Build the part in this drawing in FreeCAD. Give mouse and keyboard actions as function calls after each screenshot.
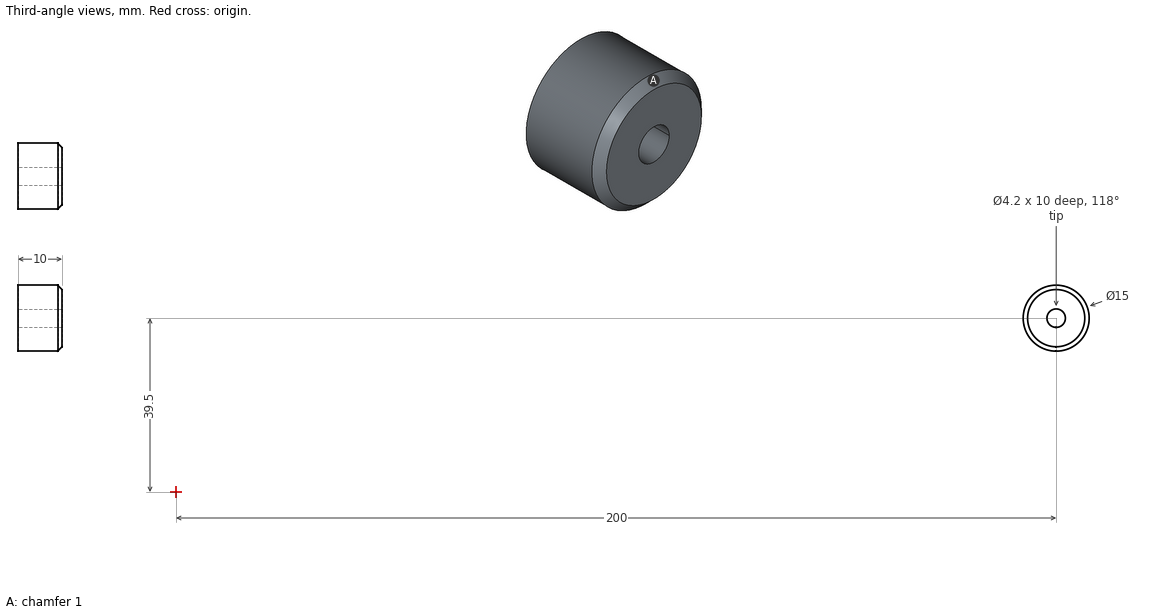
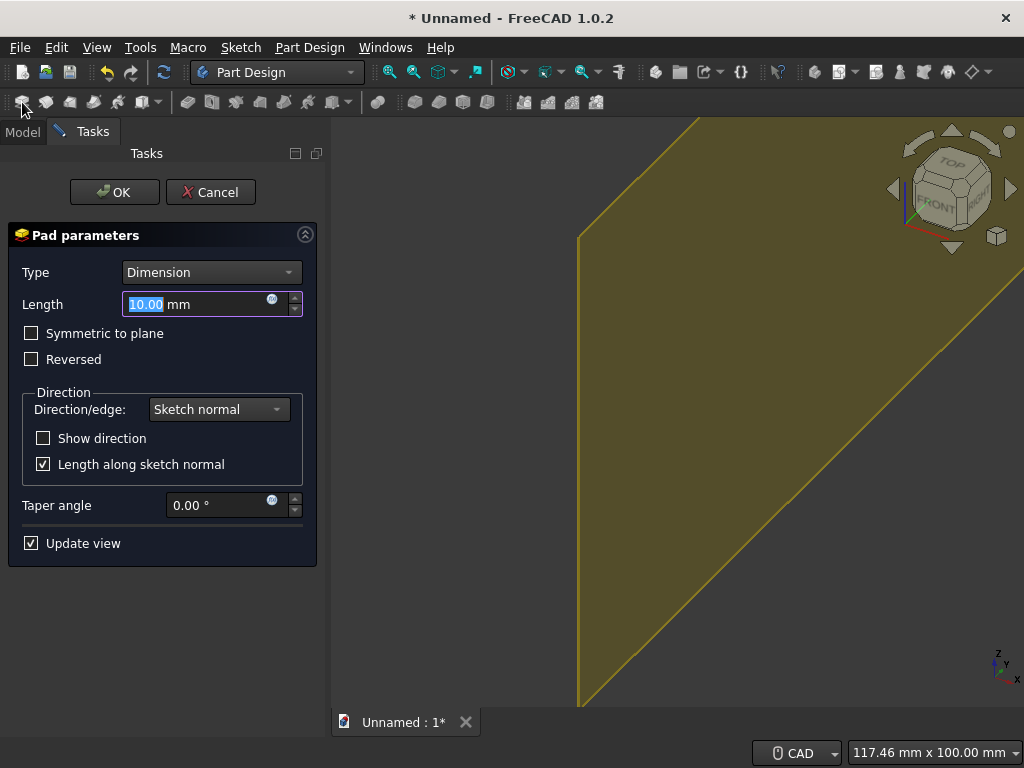
text(10)
key(Tab)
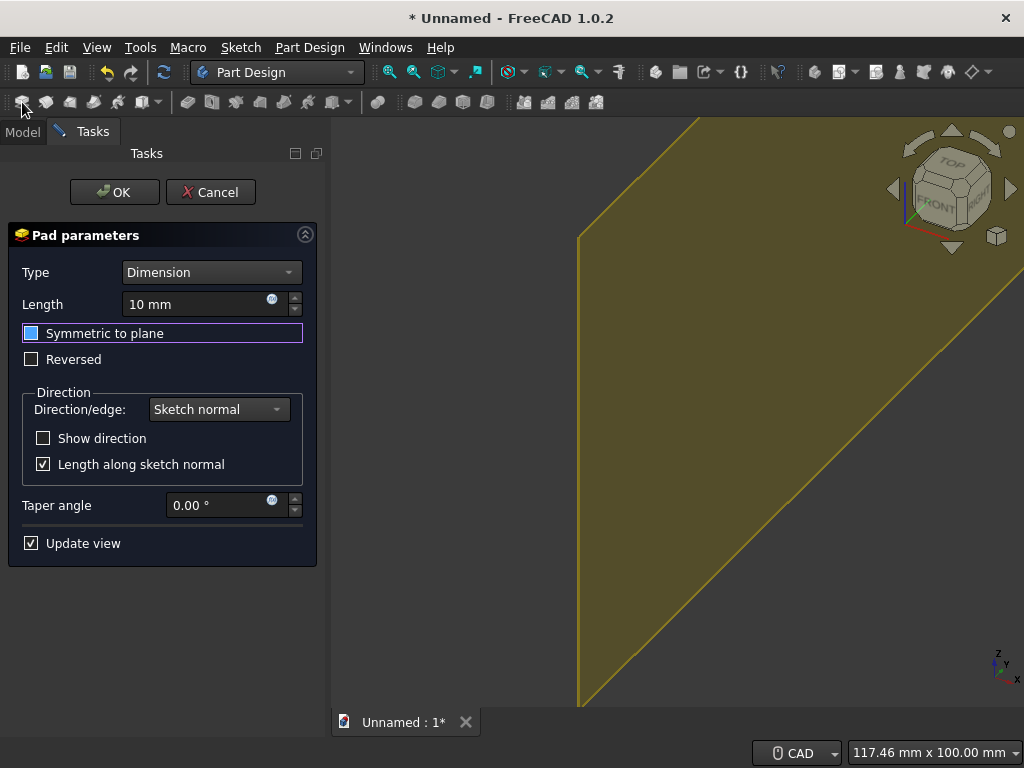
click(115, 192)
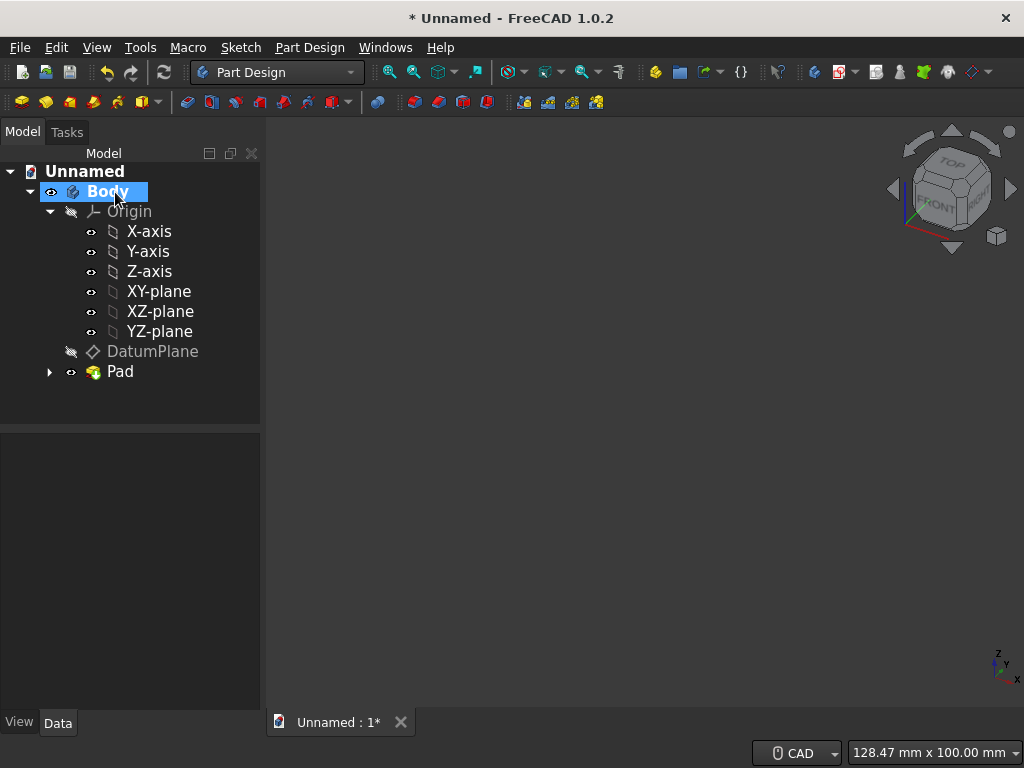
click(390, 72)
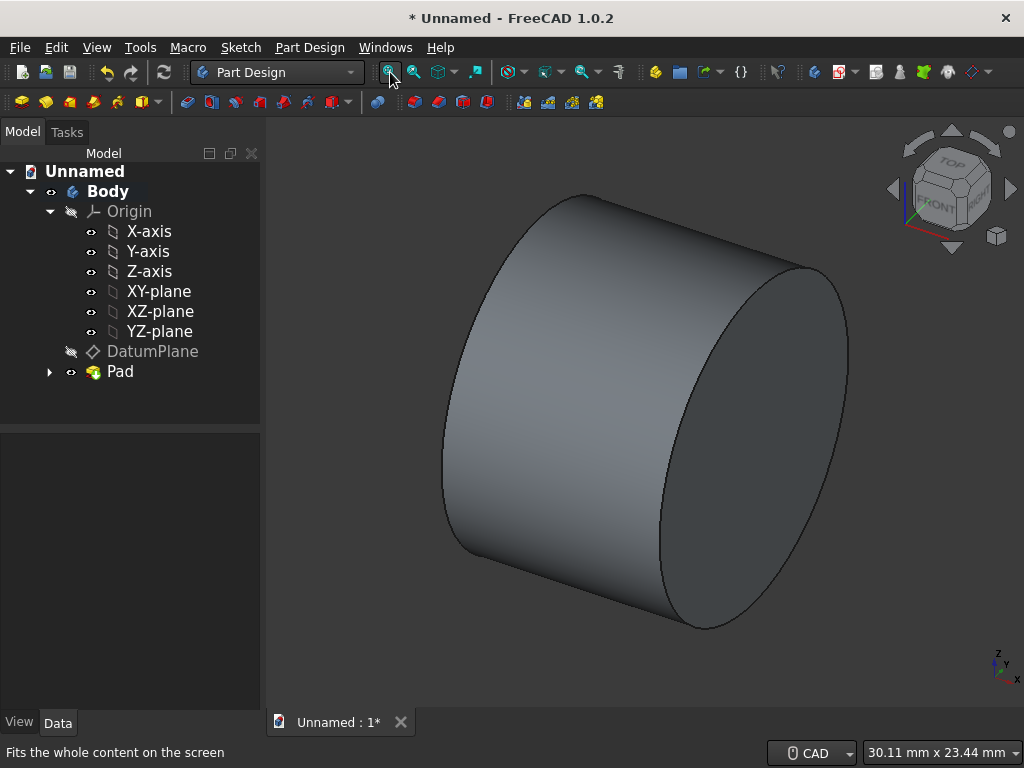
click(660, 541)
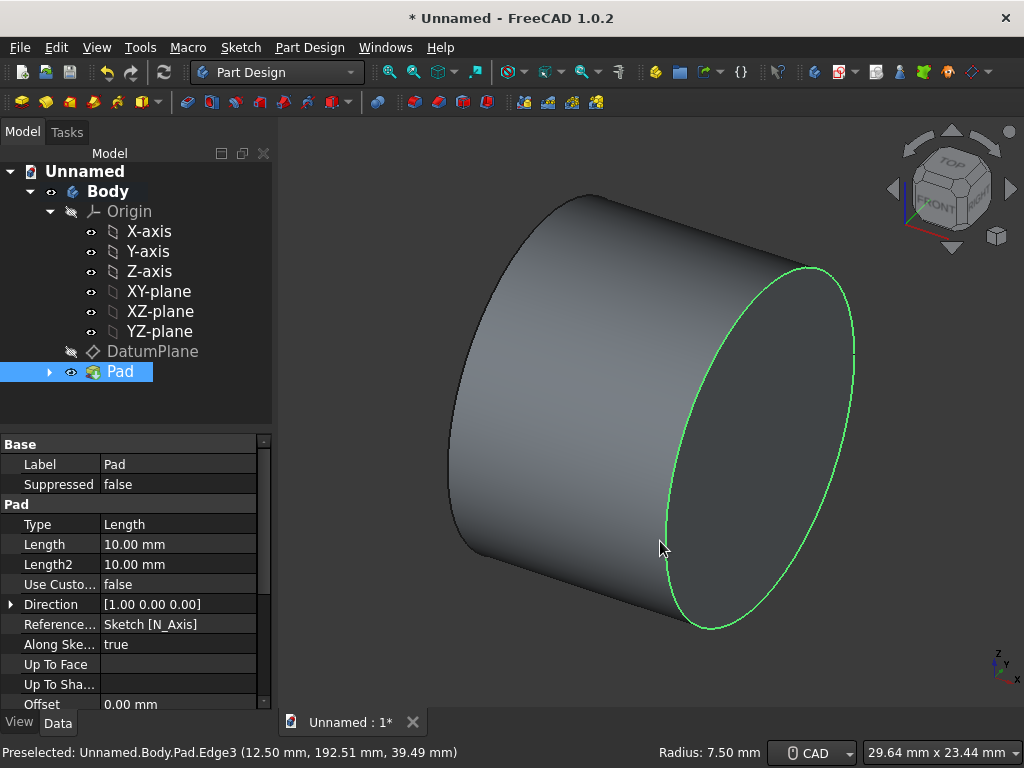
click(440, 102)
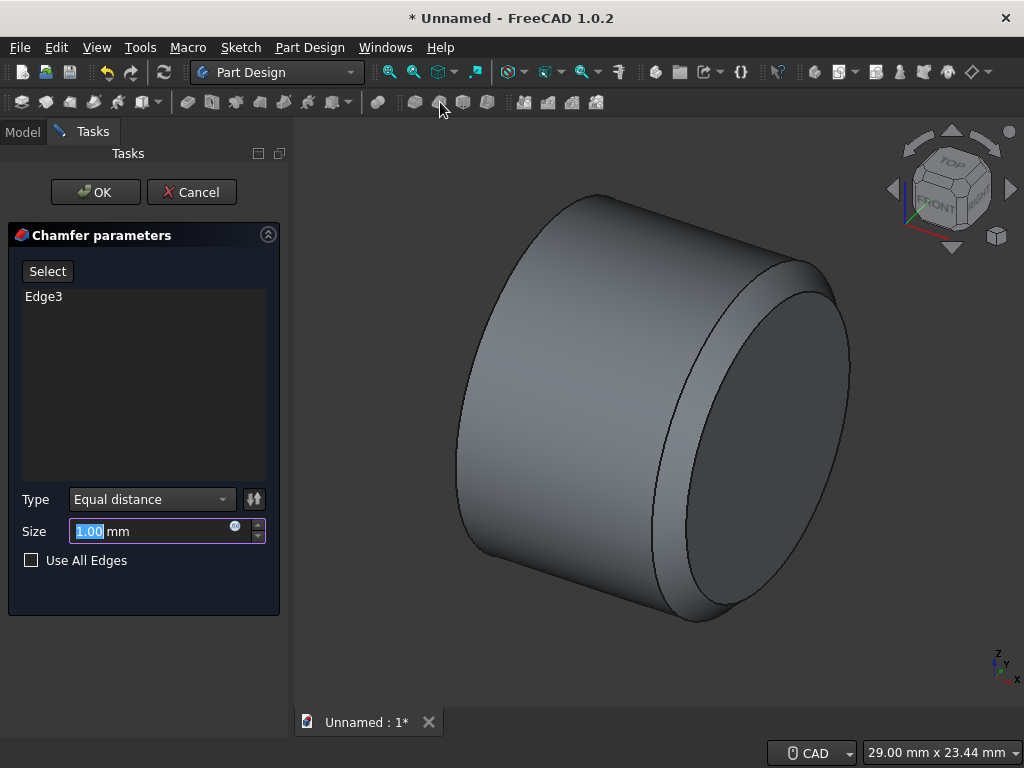
text(1)
key(Tab)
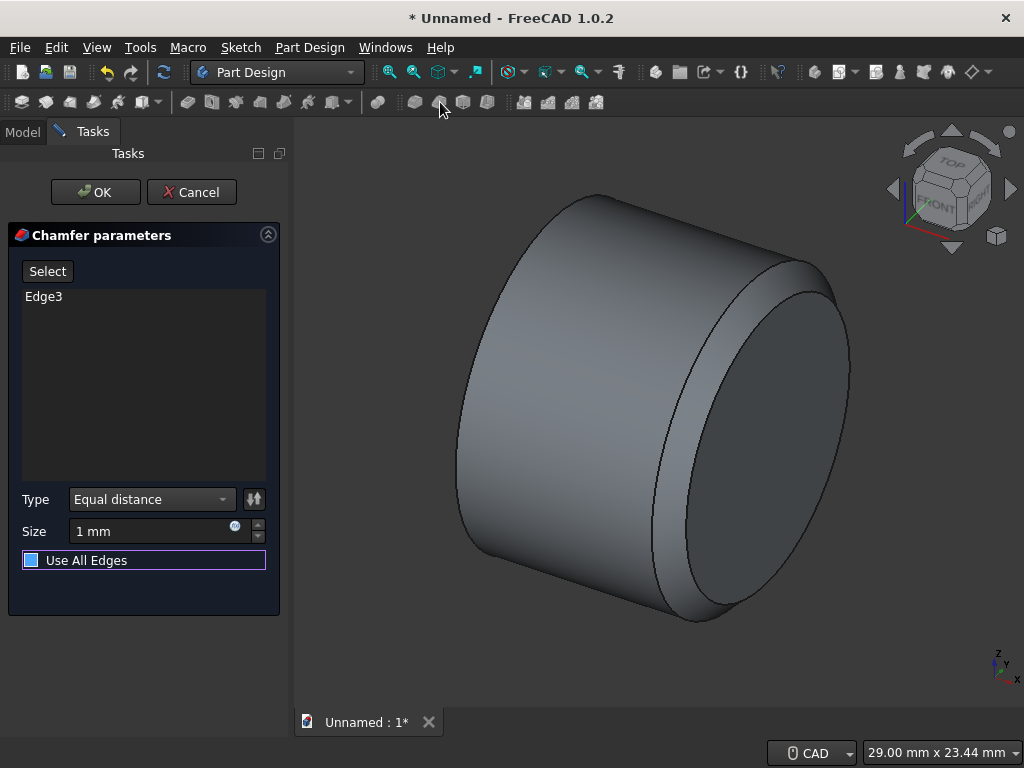
click(96, 192)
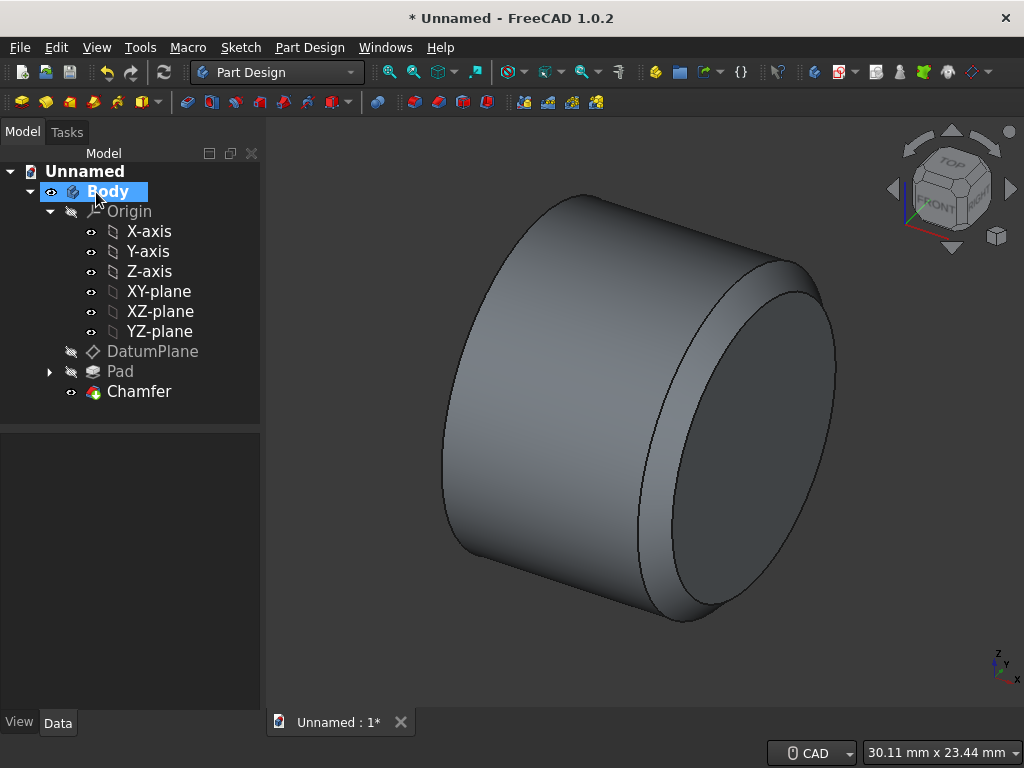
click(754, 447)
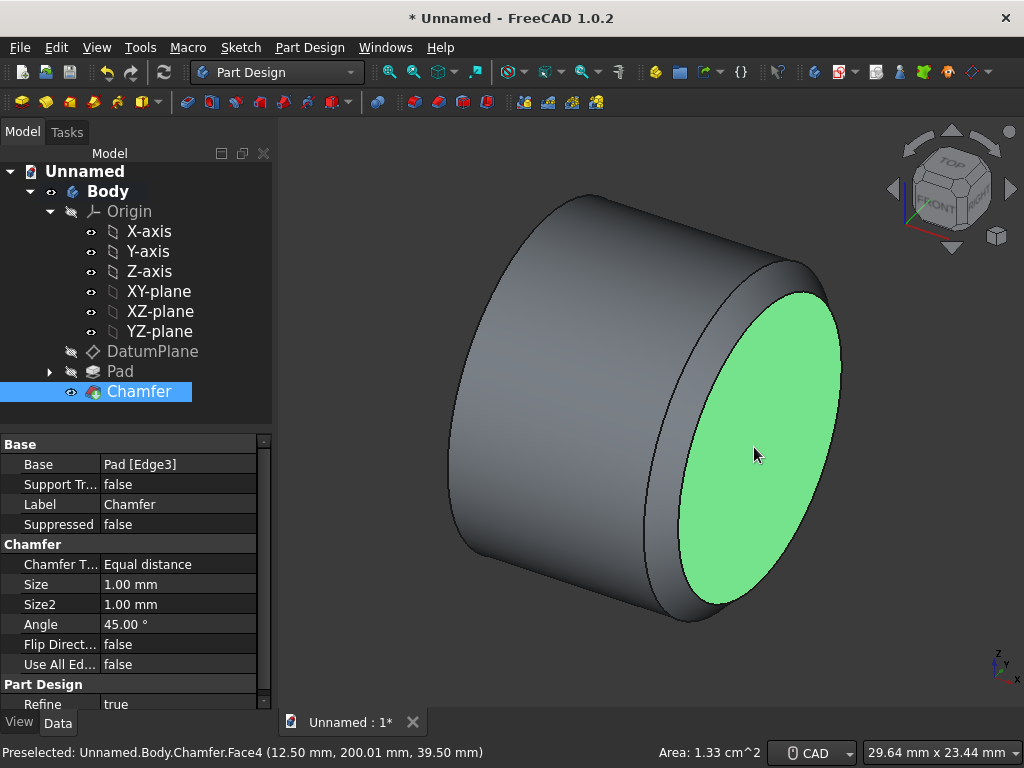
click(840, 72)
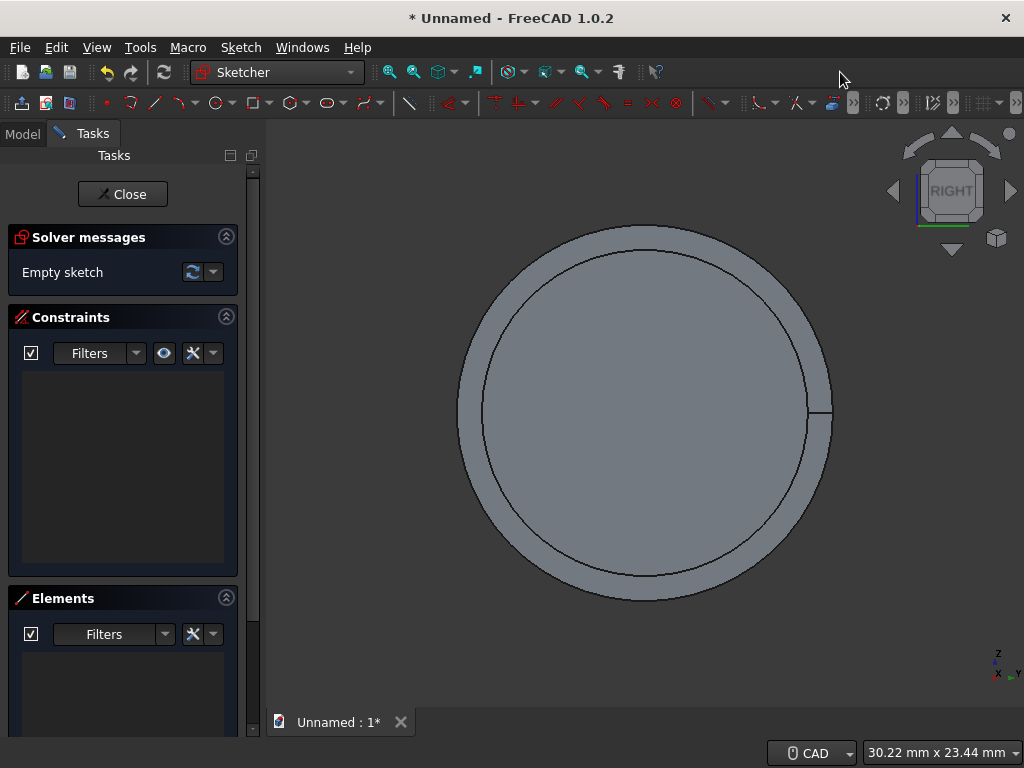
scroll(674, 413, up, 6)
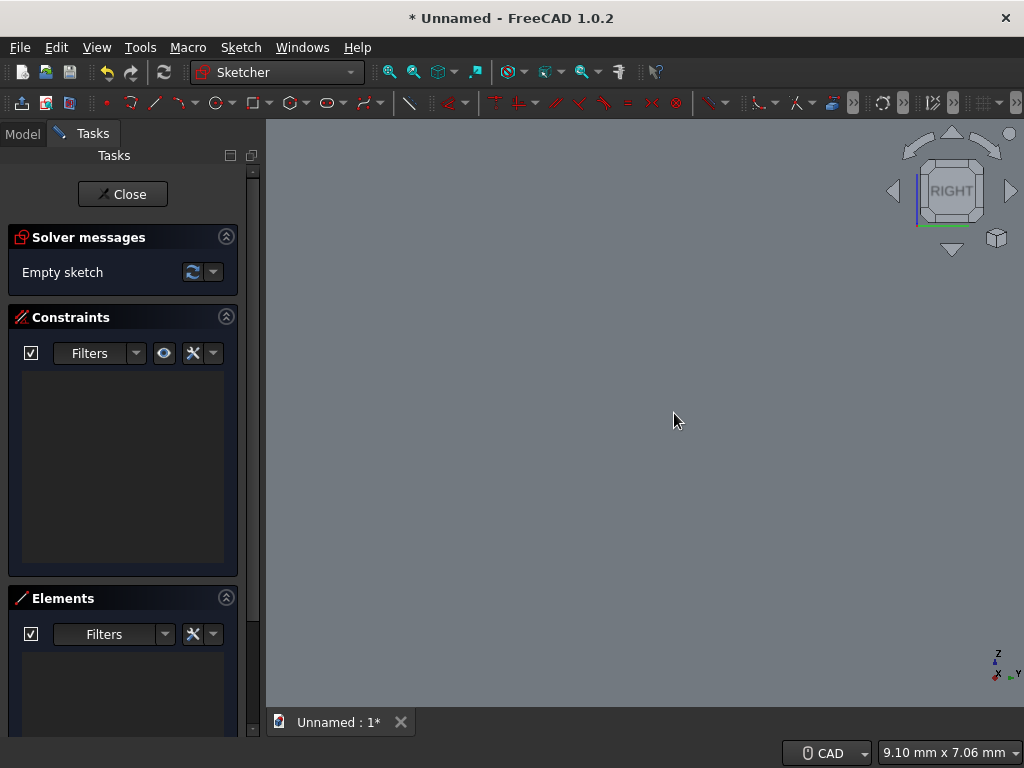
key(g)
key(c)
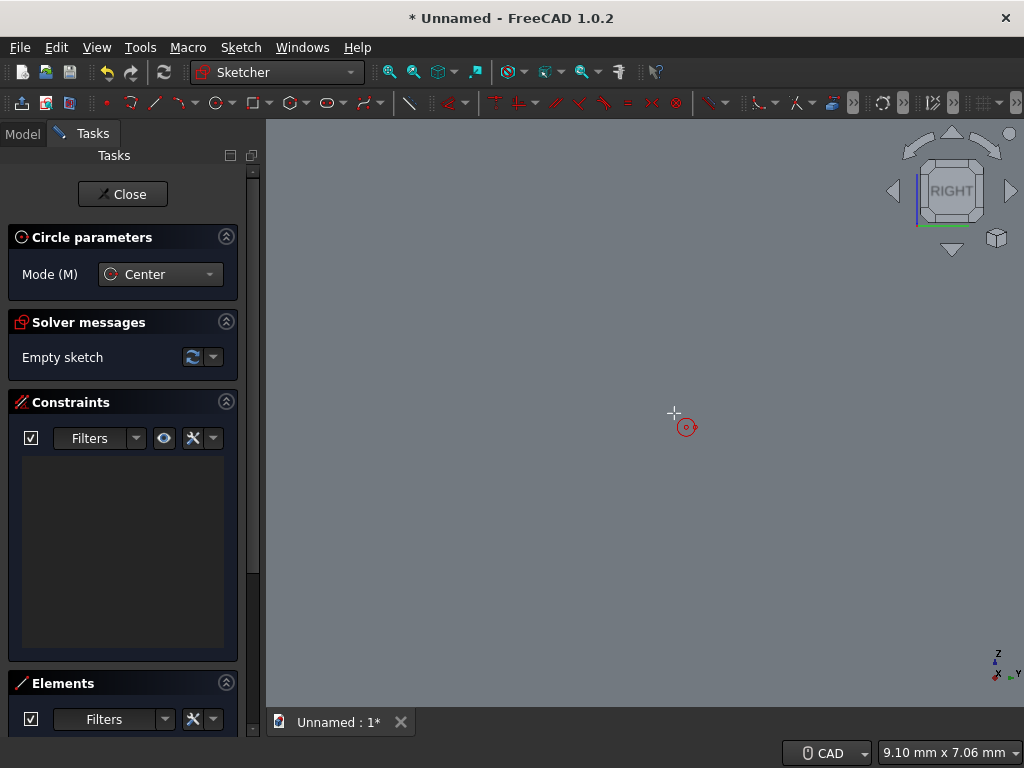
click(576, 412)
move(700, 288)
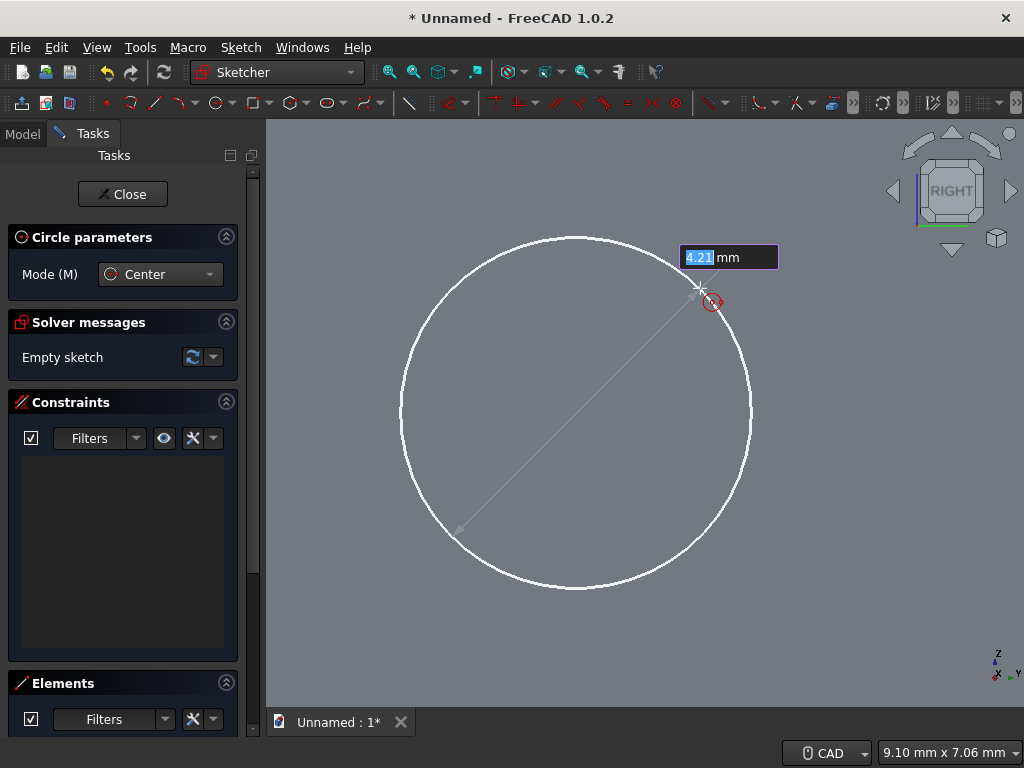
text(4.2)
key(Return)
key(Escape)